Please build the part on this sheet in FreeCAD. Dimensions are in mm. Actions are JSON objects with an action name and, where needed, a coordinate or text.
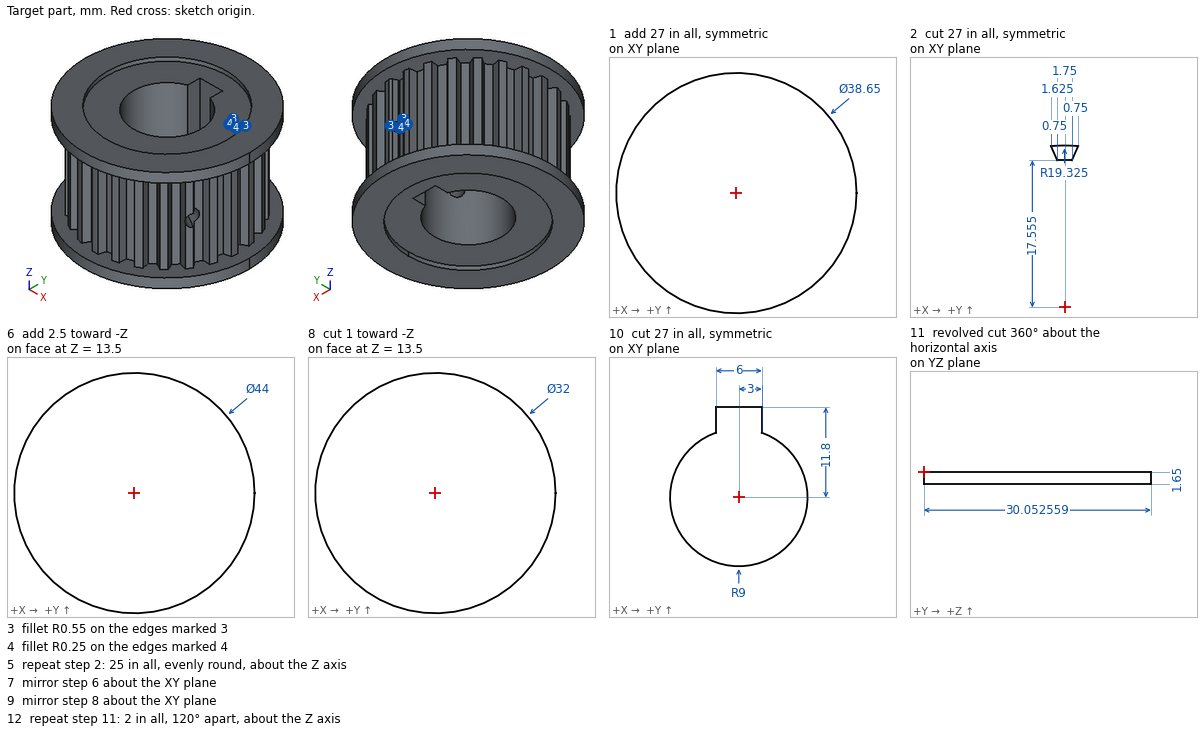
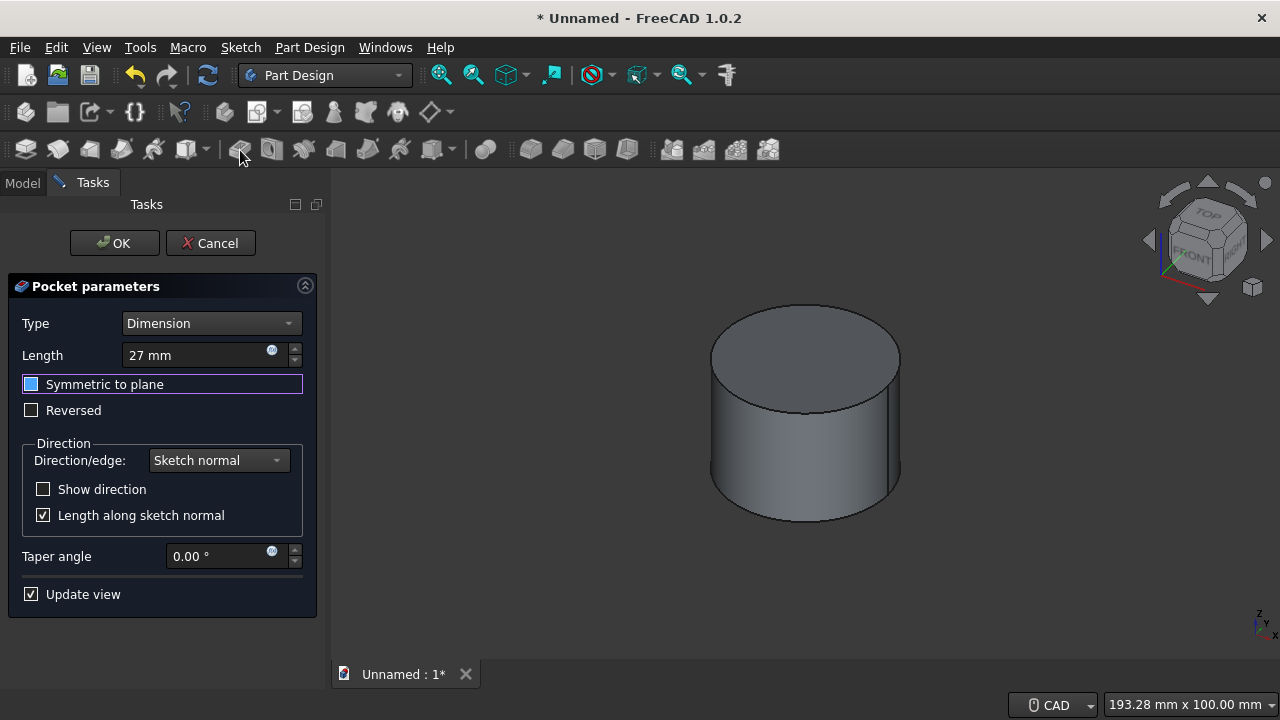
{"action": "left_click", "coordinate": [30, 384]}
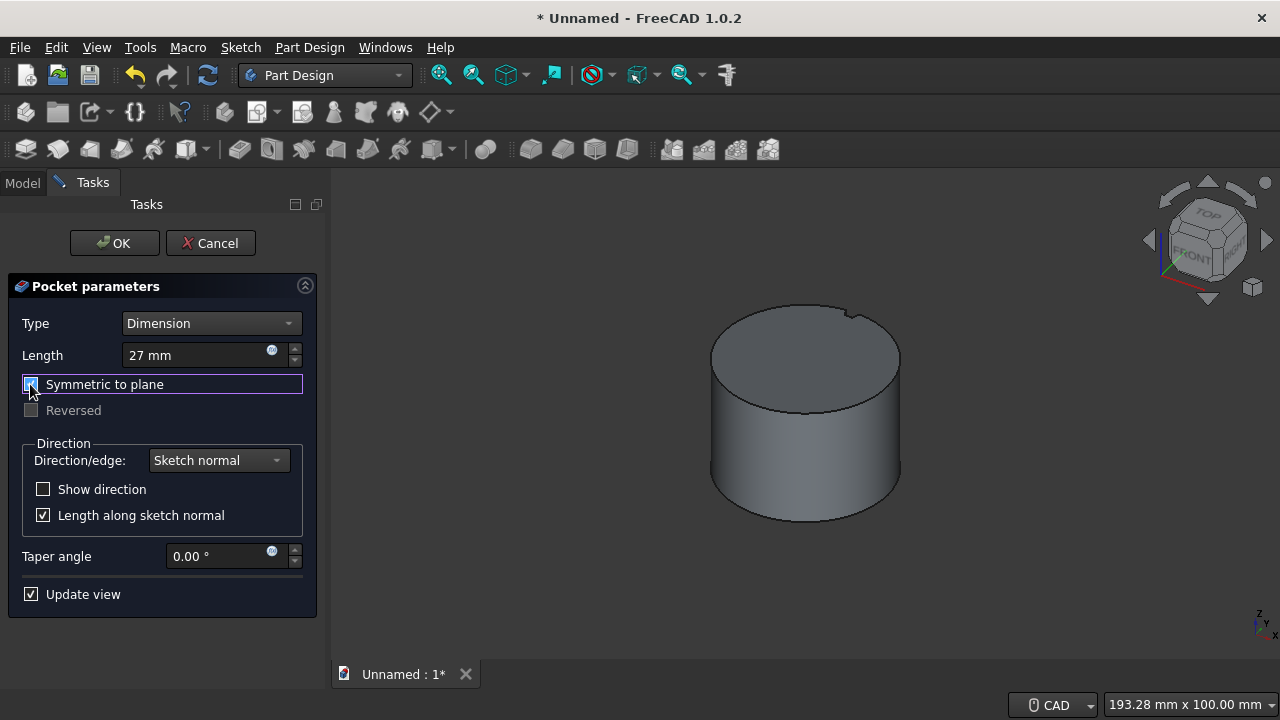
{"action": "left_click", "coordinate": [115, 243]}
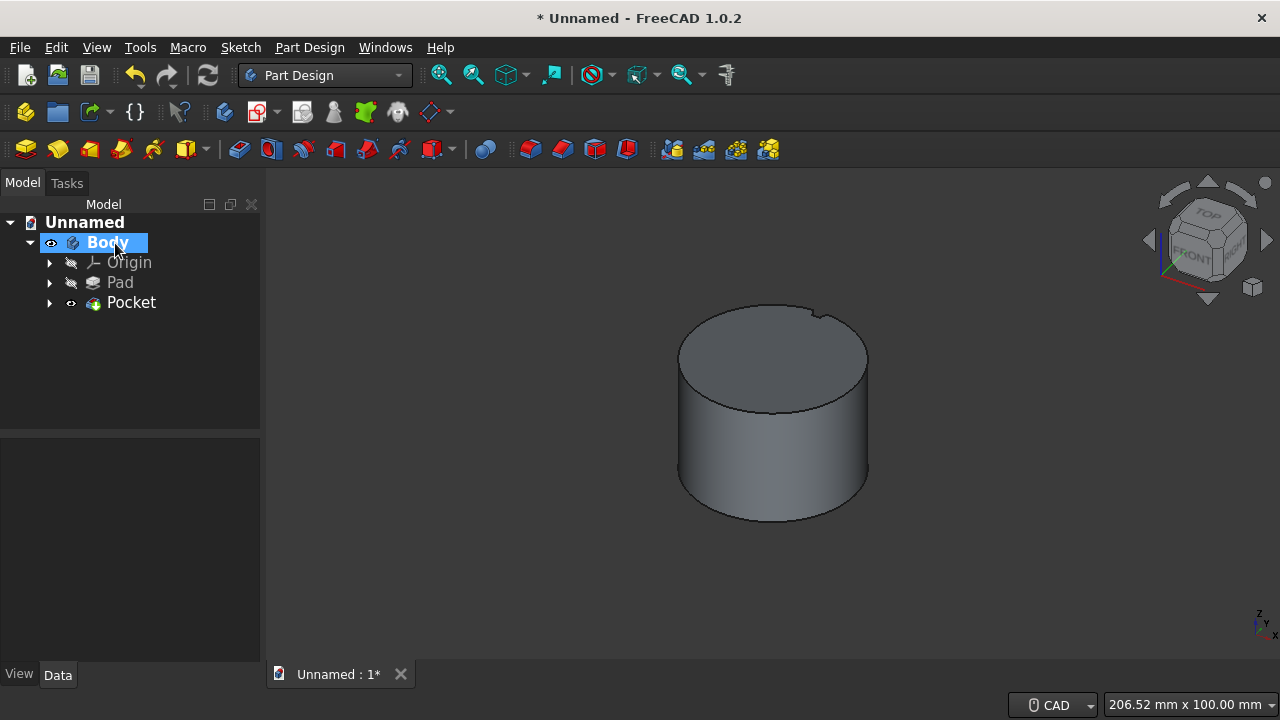
{"action": "key", "text": "0"}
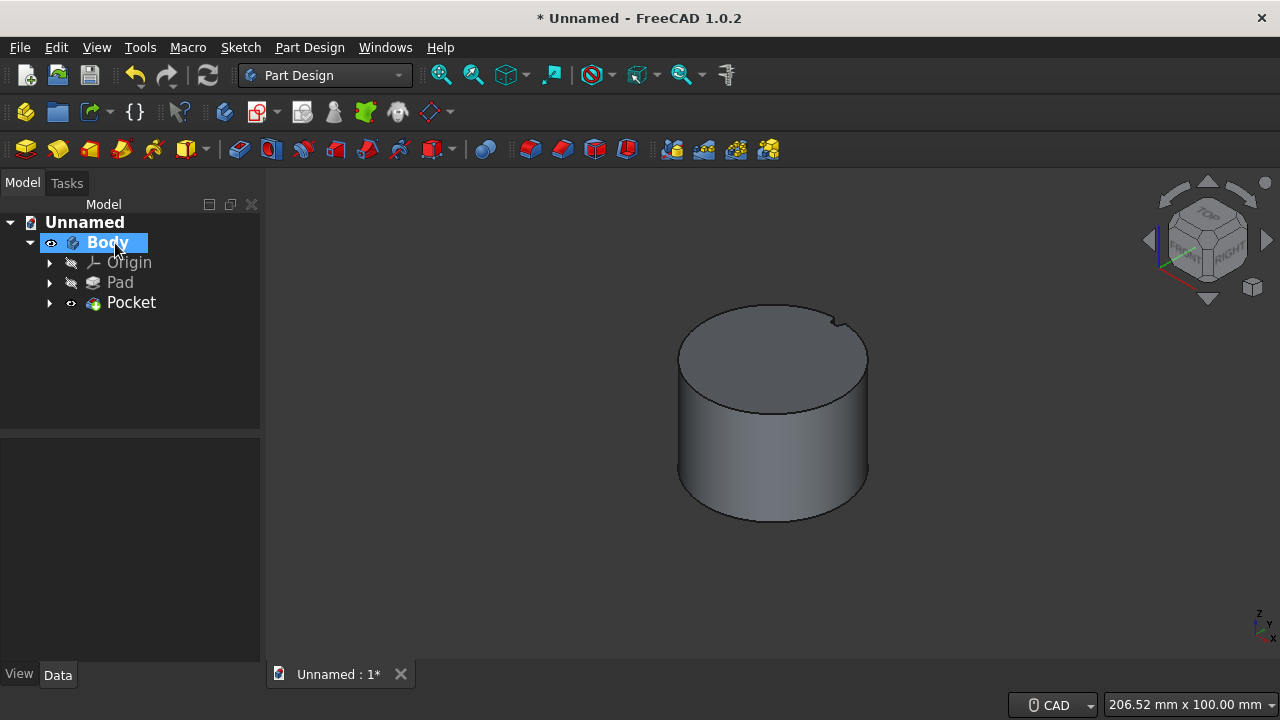
{"action": "key", "text": "2"}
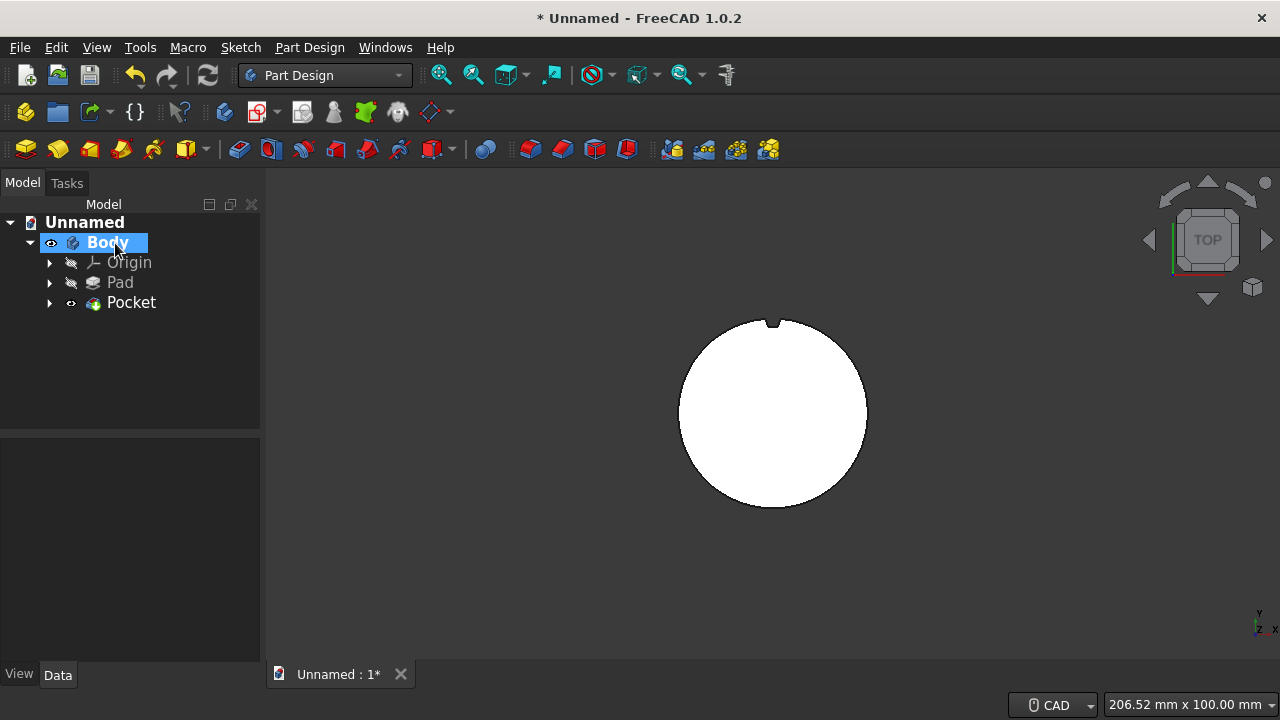
{"action": "left_click", "coordinate": [442, 76]}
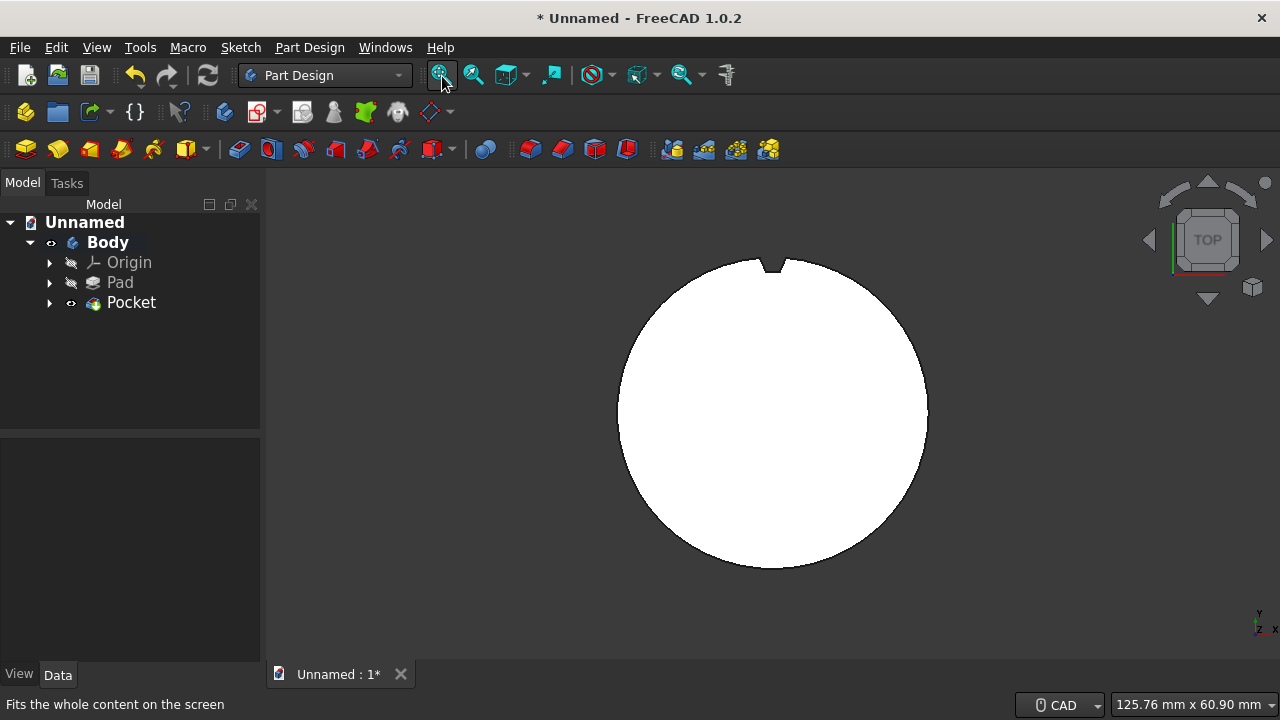
{"action": "key", "text": "1"}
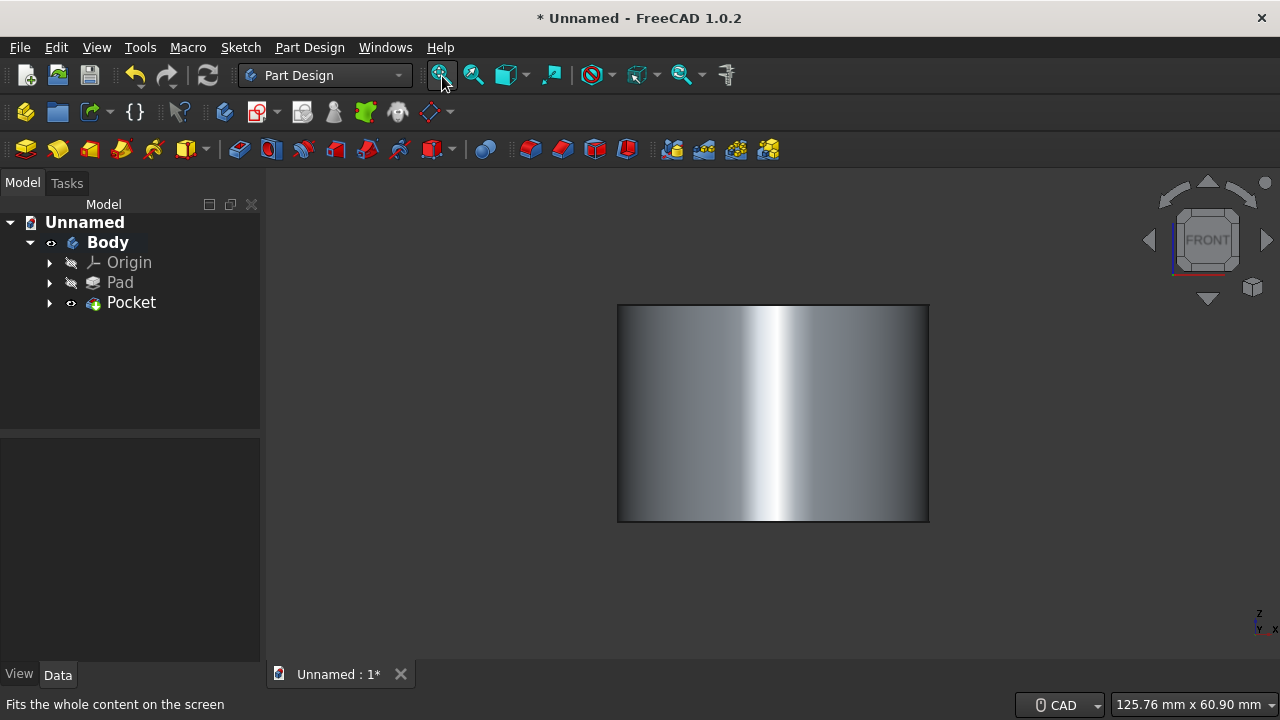
{"action": "left_click", "coordinate": [442, 76]}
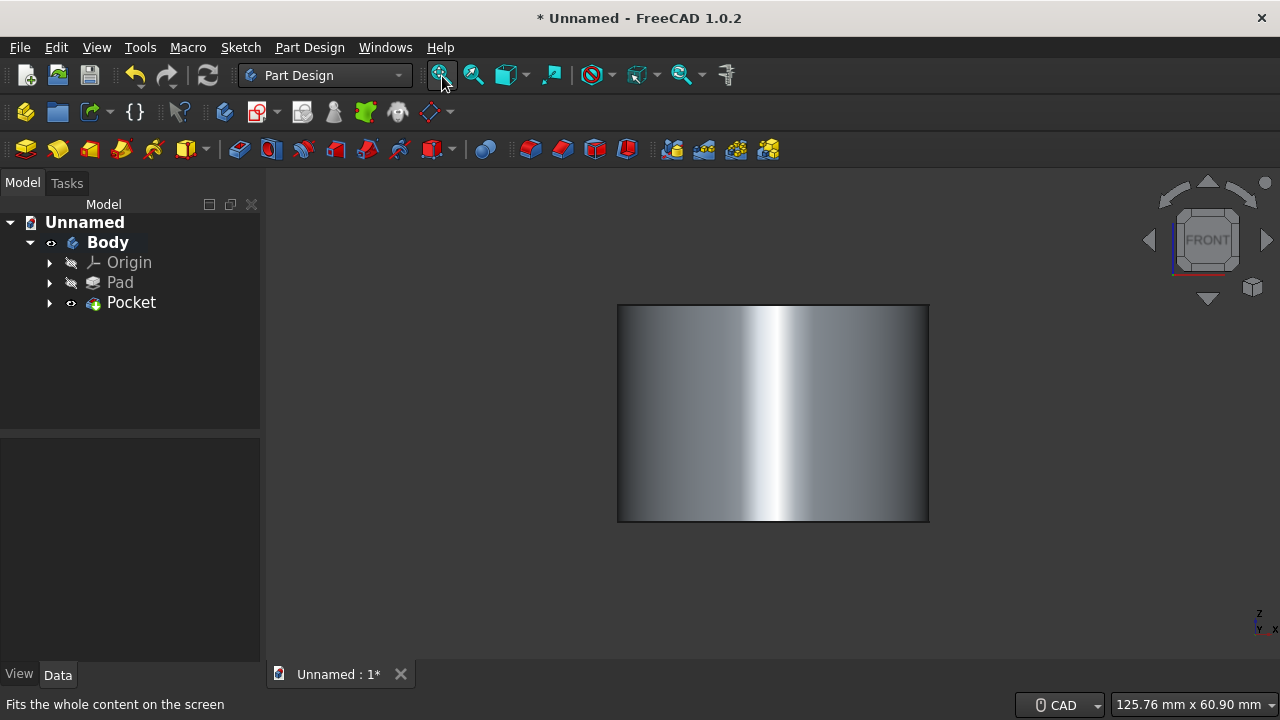
{"action": "key", "text": "3"}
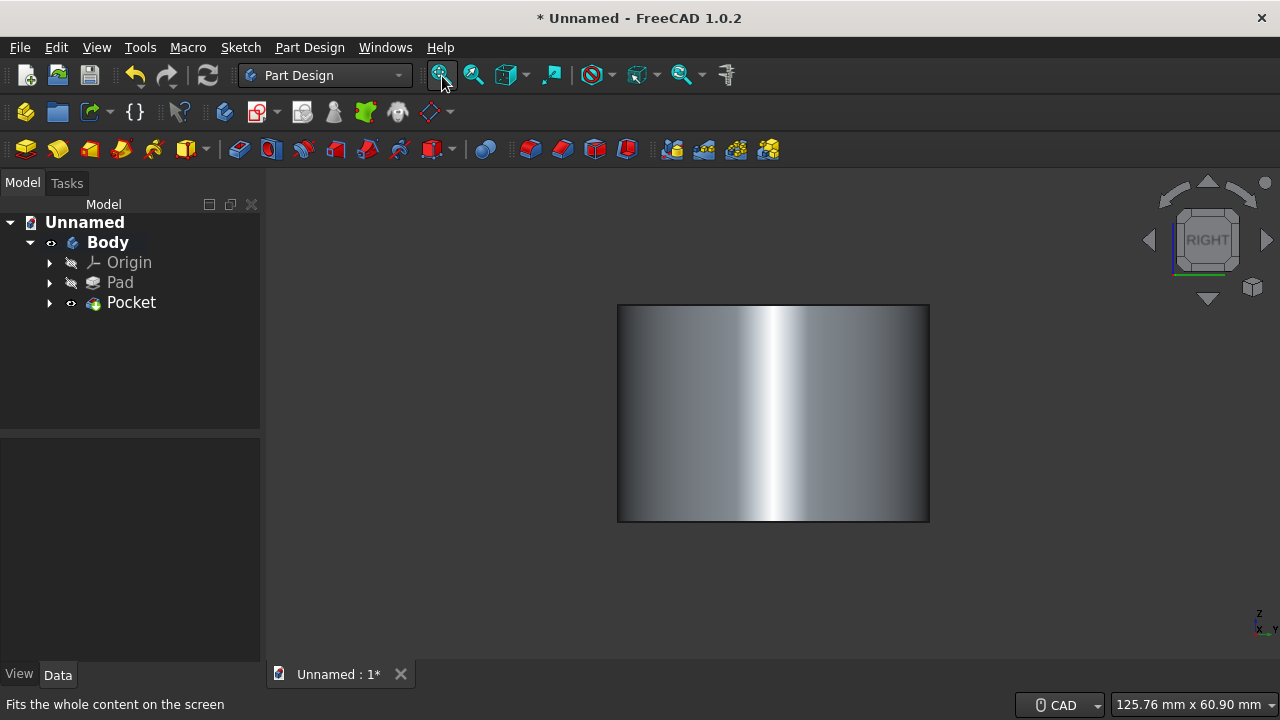
{"action": "left_click", "coordinate": [442, 76]}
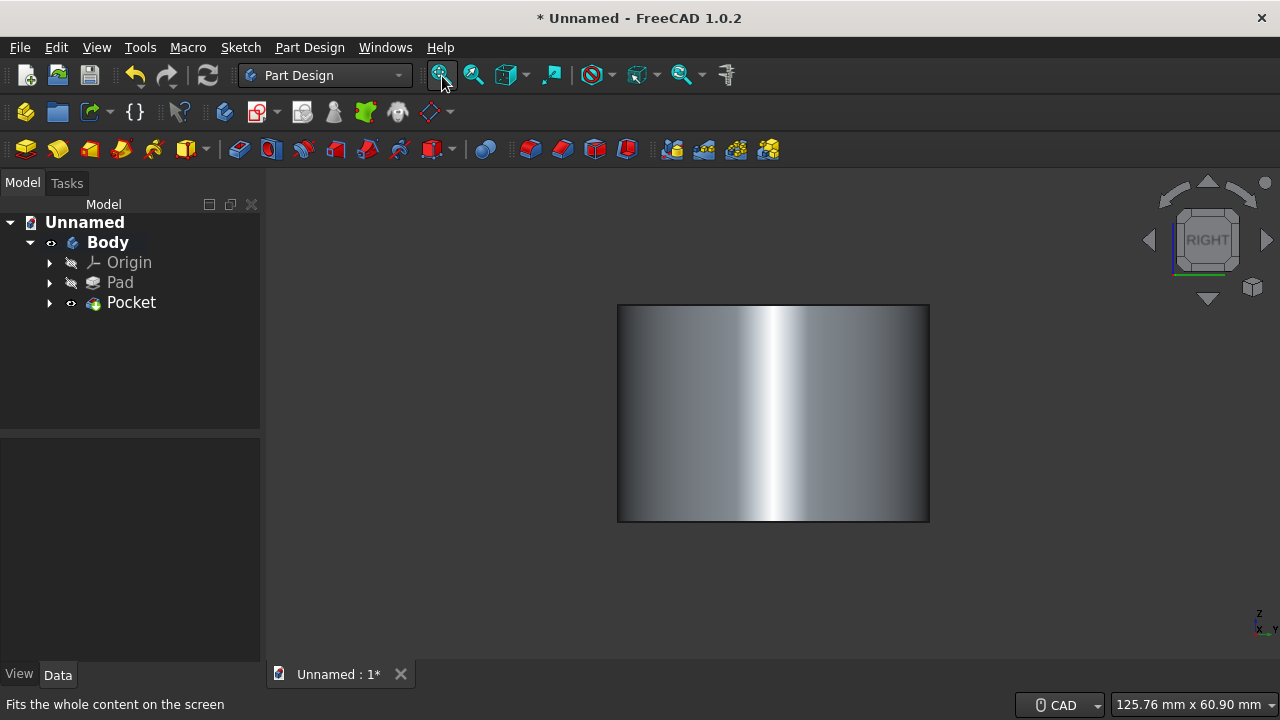
{"action": "key", "text": "5"}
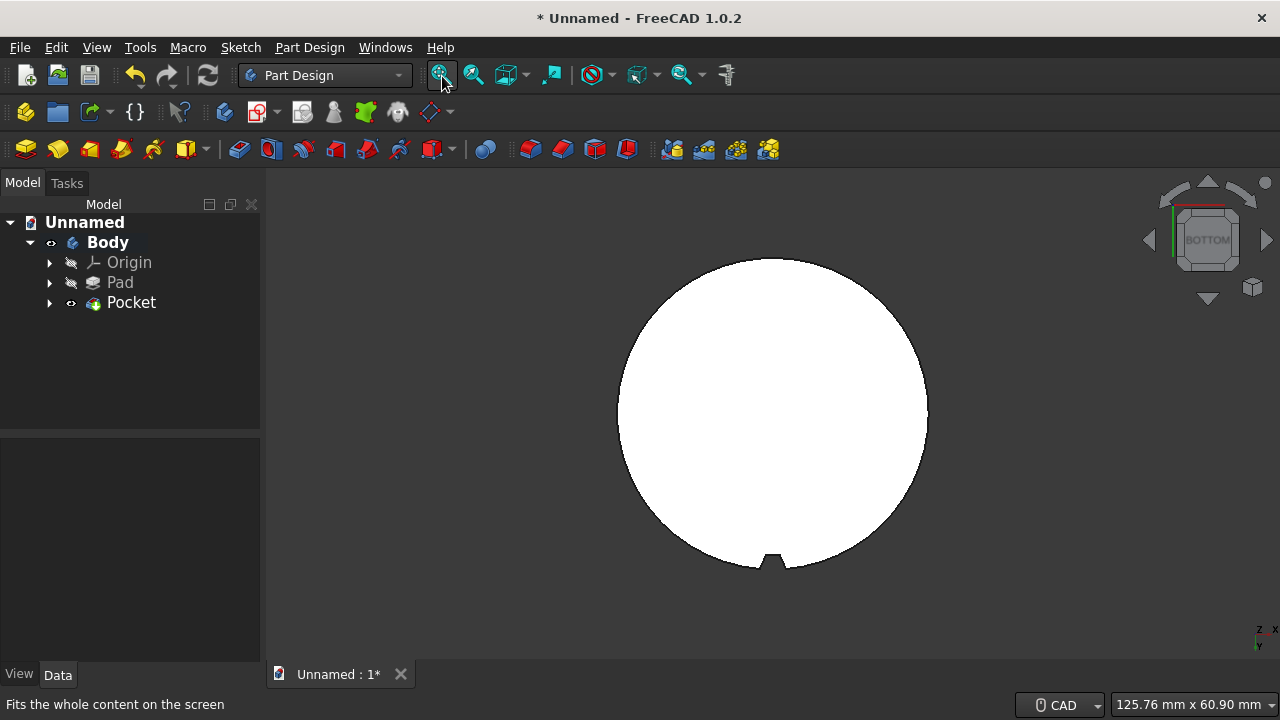
{"action": "key", "text": "4"}